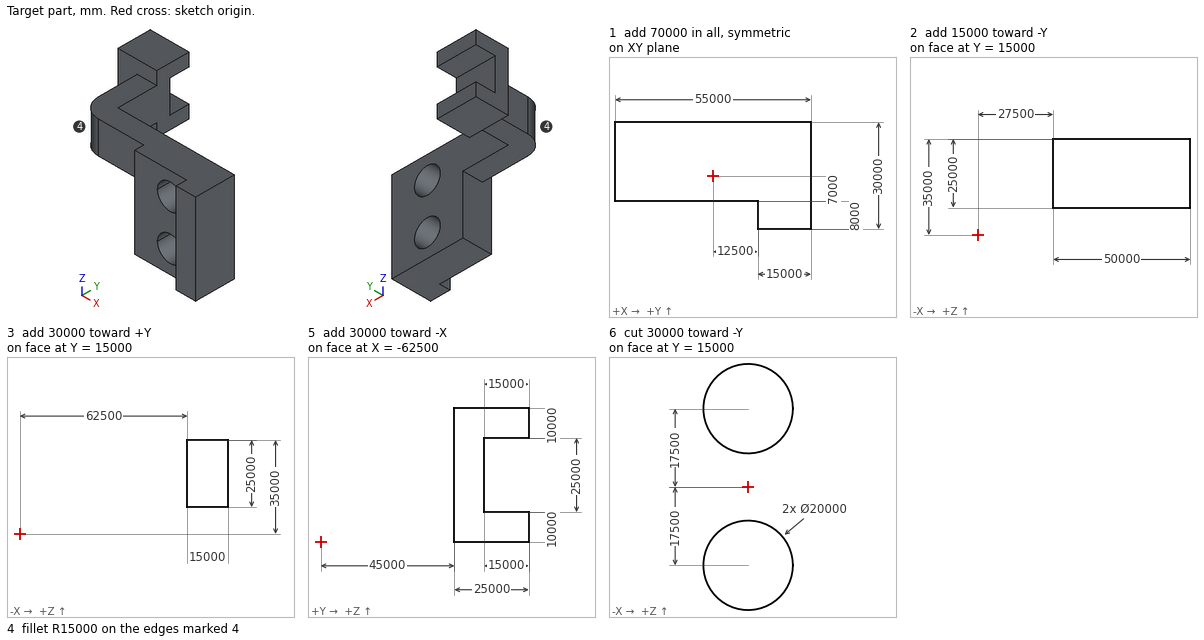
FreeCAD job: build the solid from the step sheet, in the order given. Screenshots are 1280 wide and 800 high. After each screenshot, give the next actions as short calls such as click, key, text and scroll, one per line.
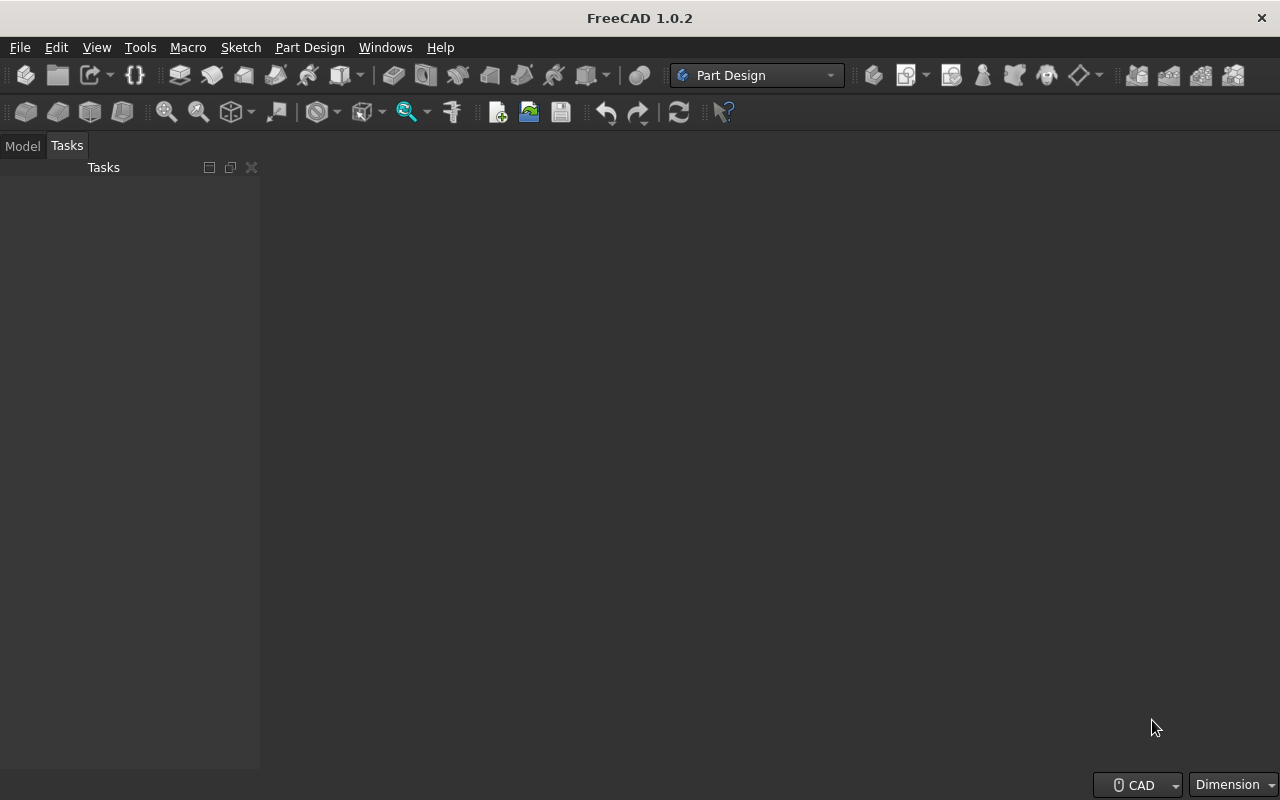
key(ctrl+n)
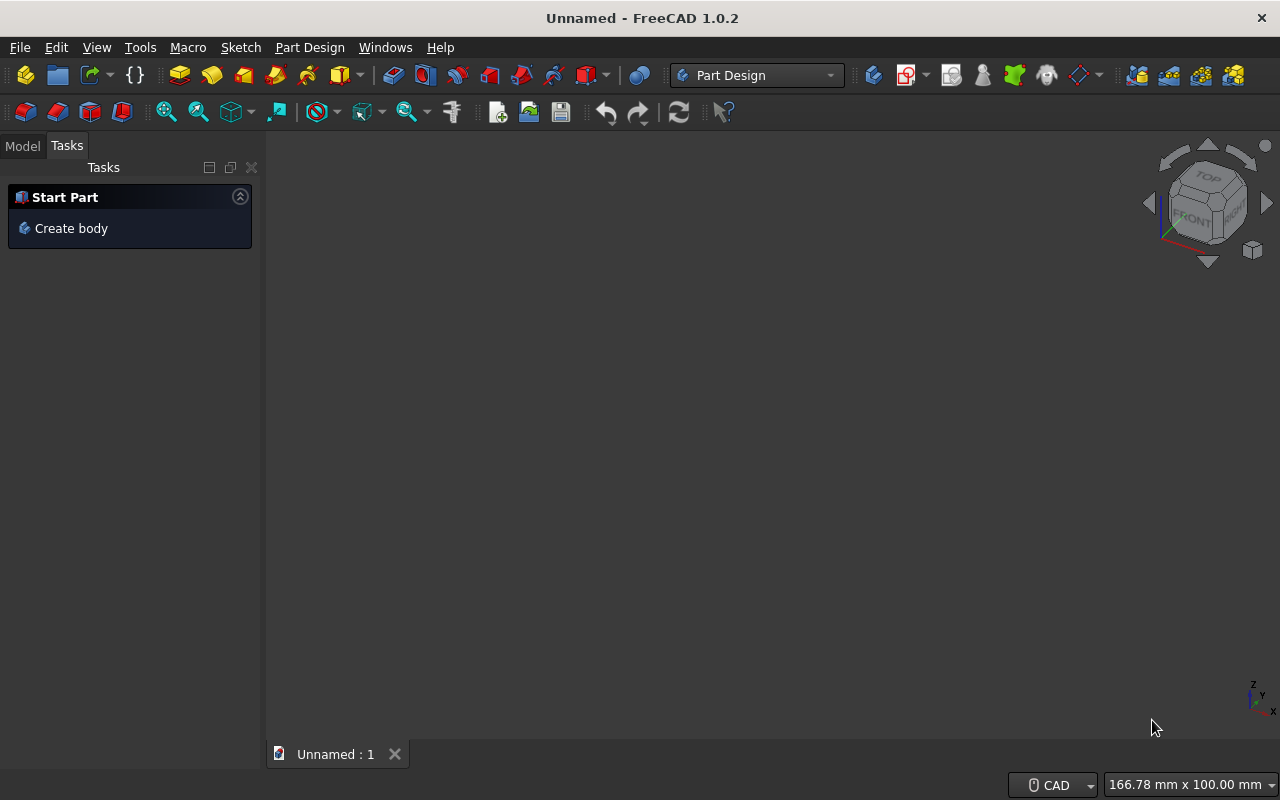
click(906, 76)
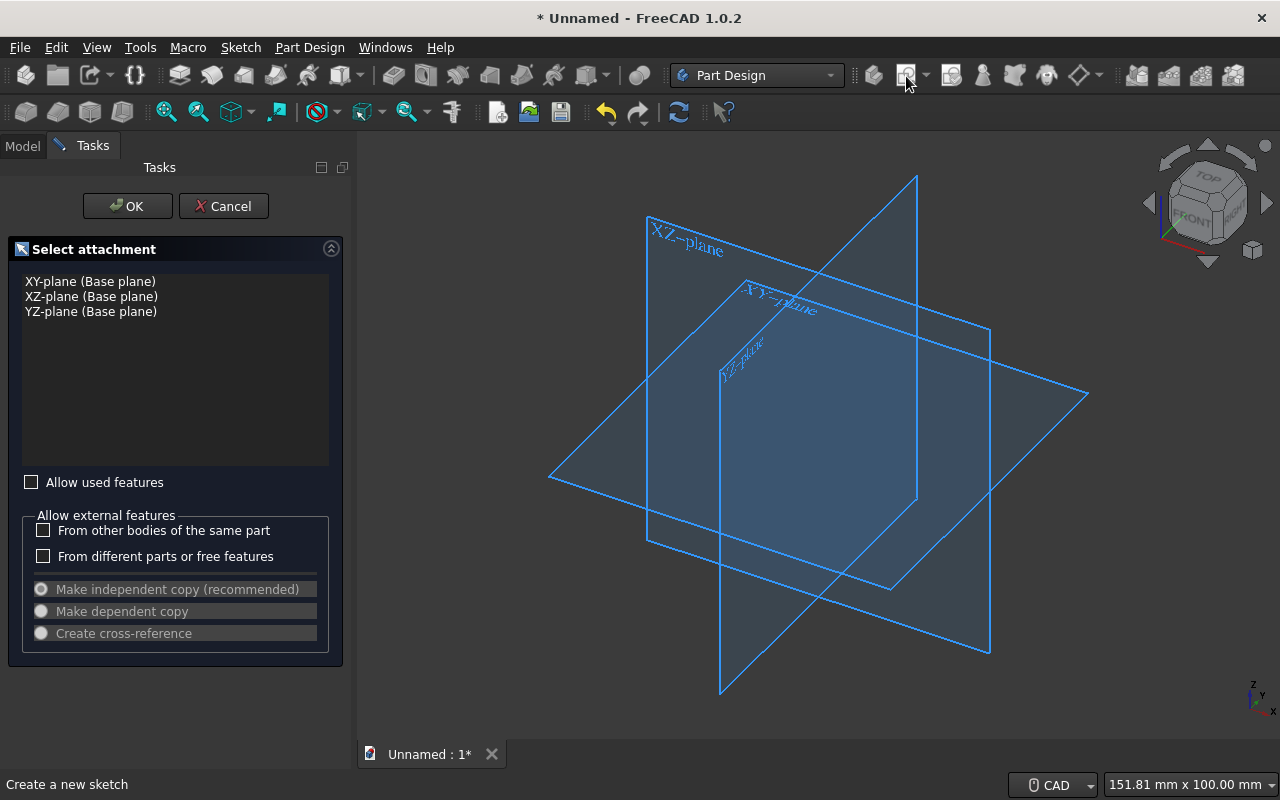
click(82, 282)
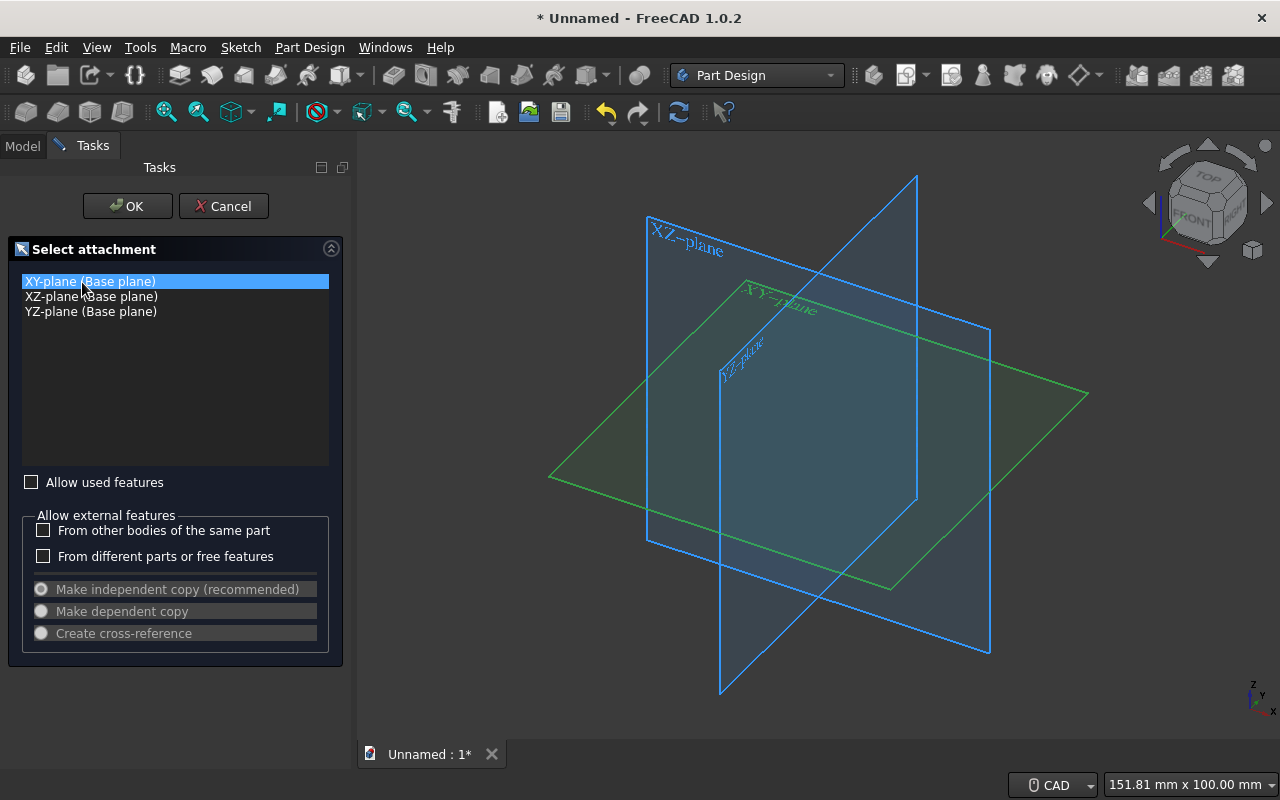
click(128, 206)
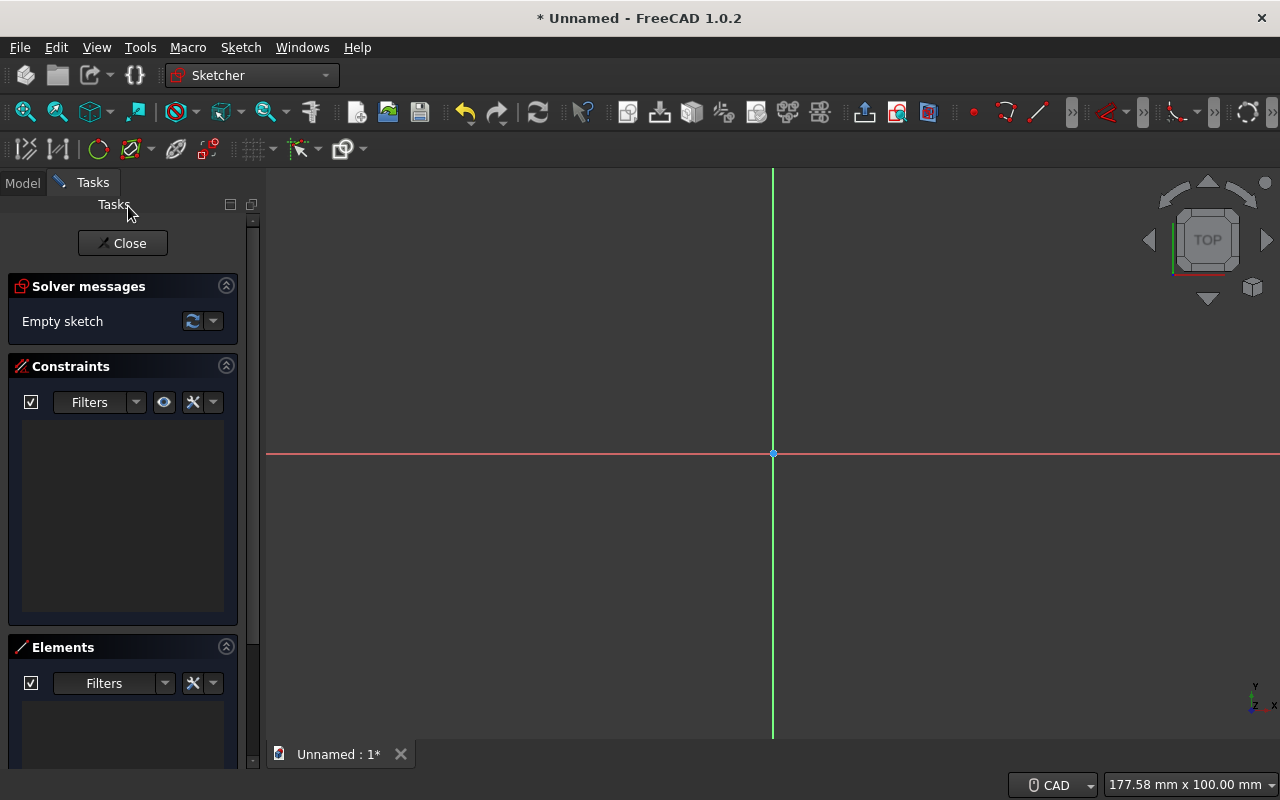
scroll(704, 454, down, 15)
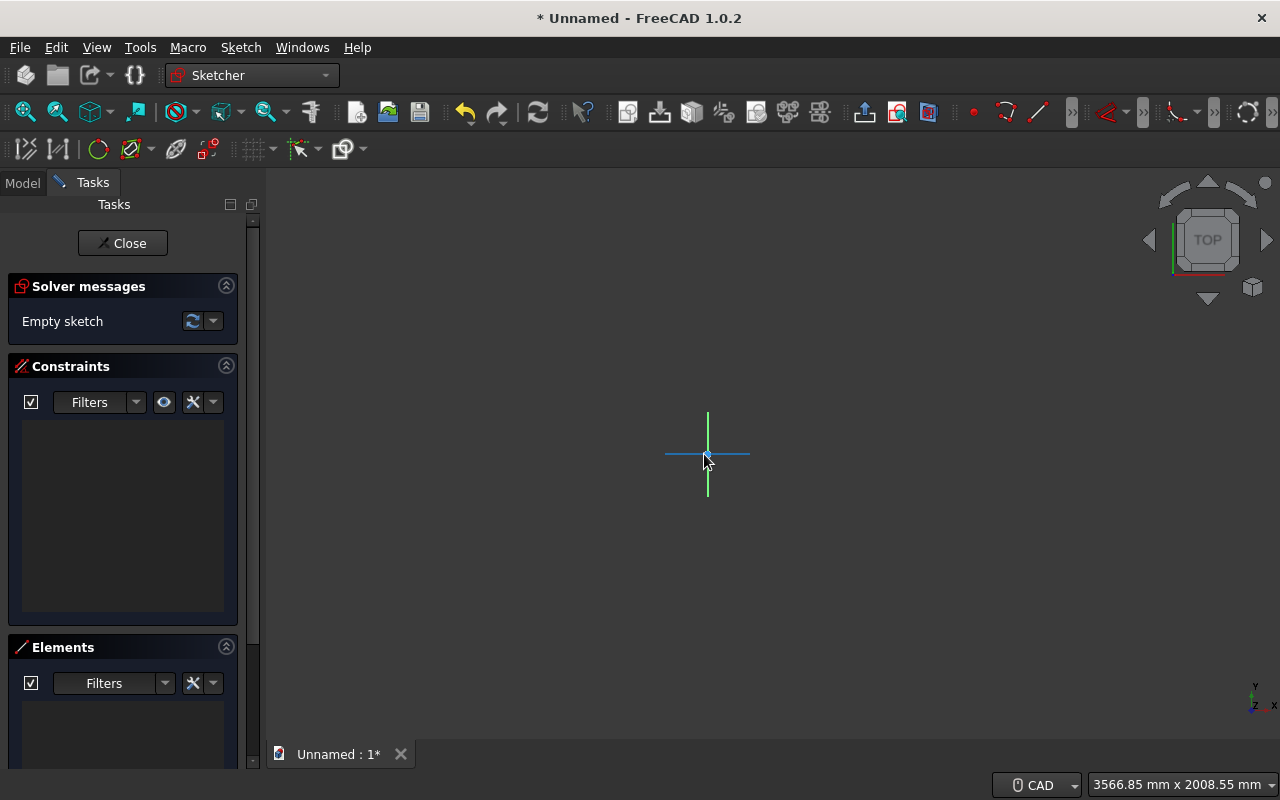
scroll(704, 453, down, 16)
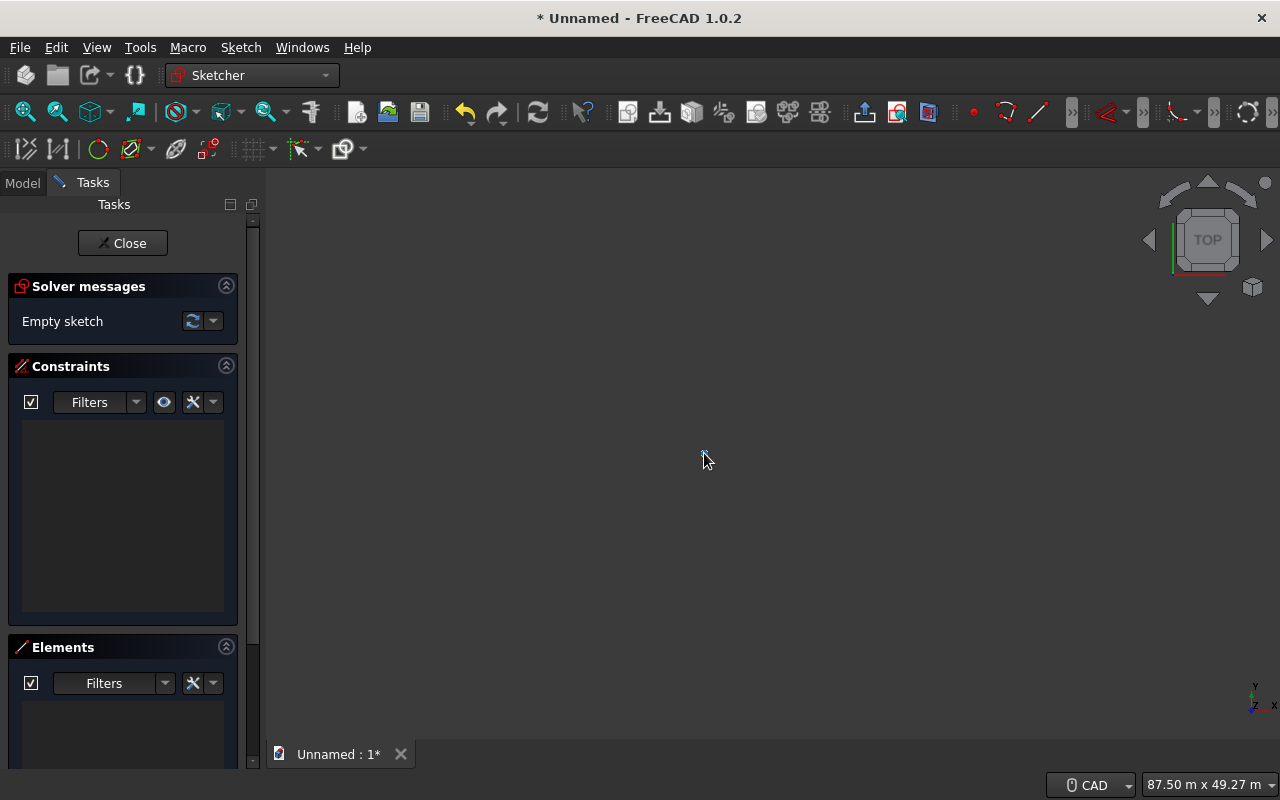
click(1006, 112)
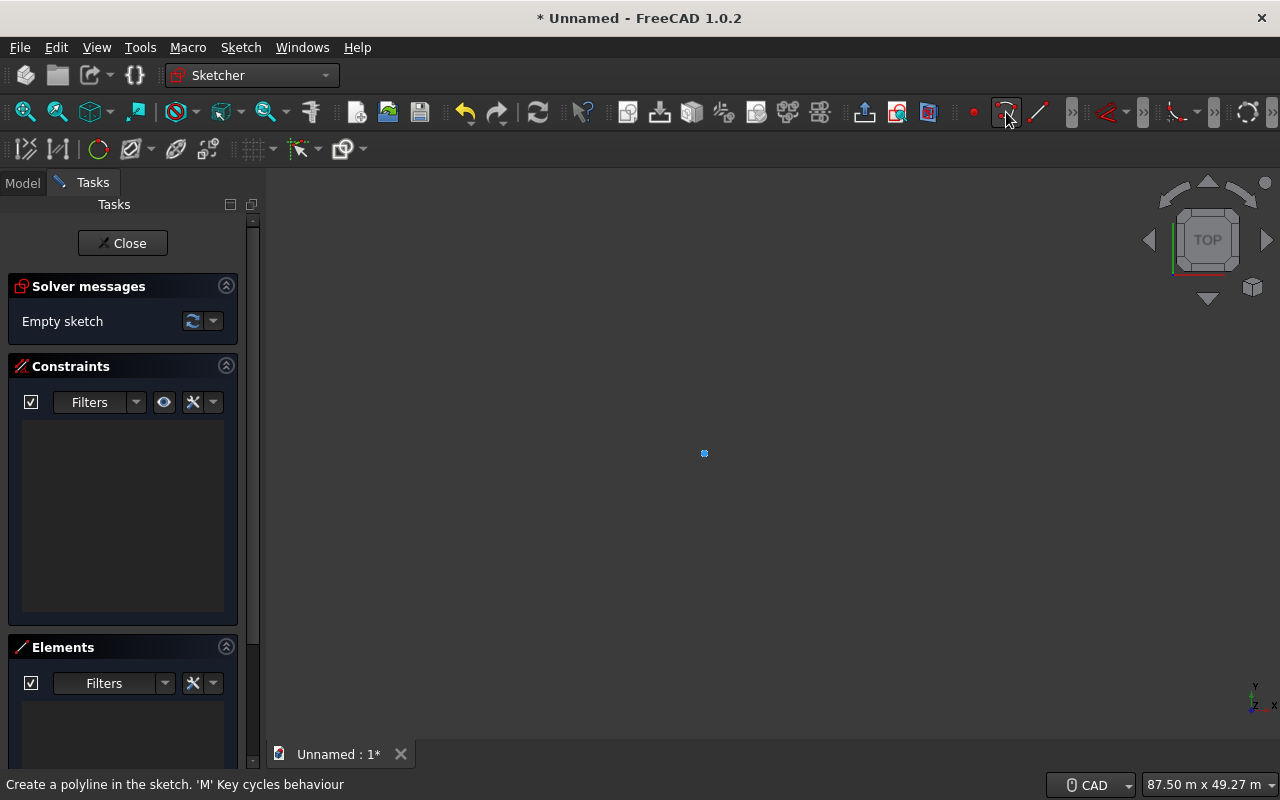
click(849, 535)
click(849, 627)
click(1023, 627)
click(1023, 280)
click(386, 280)
click(386, 535)
click(849, 536)
key(Escape)
key(Escape)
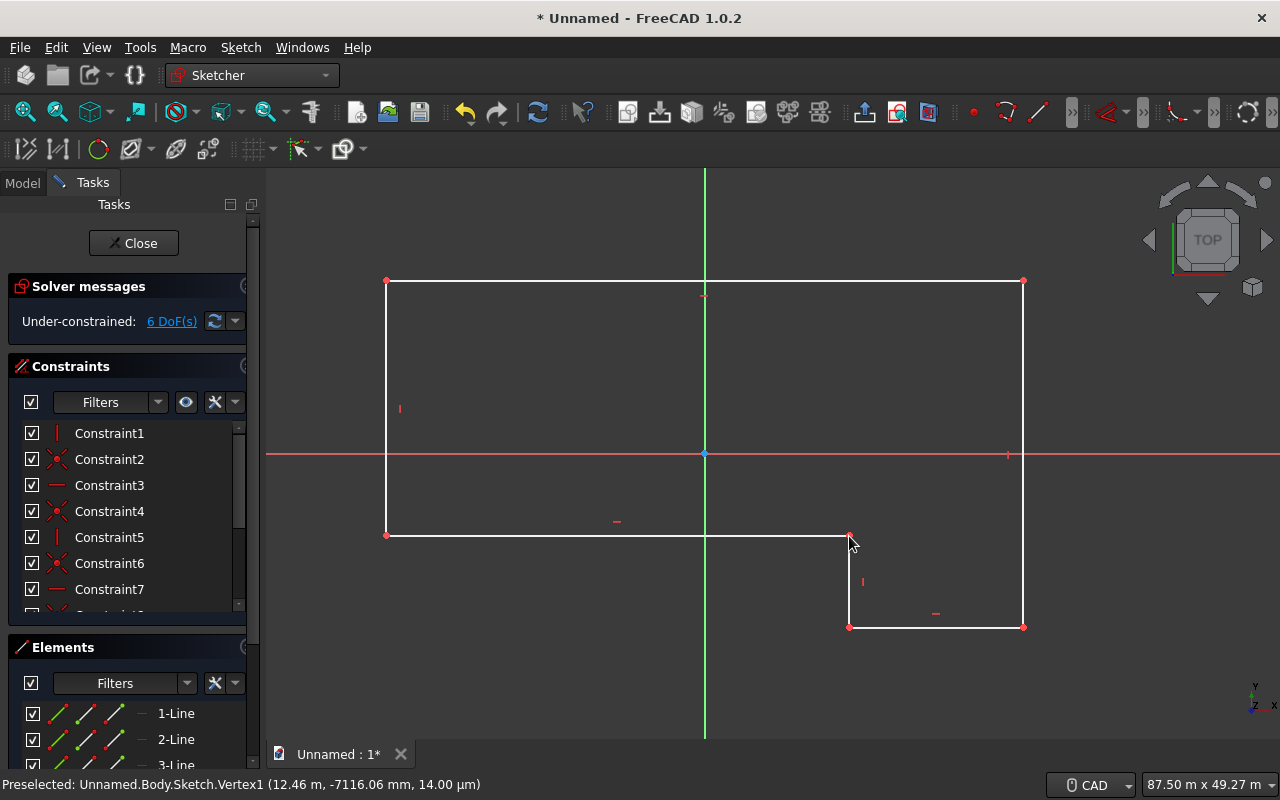
key(d)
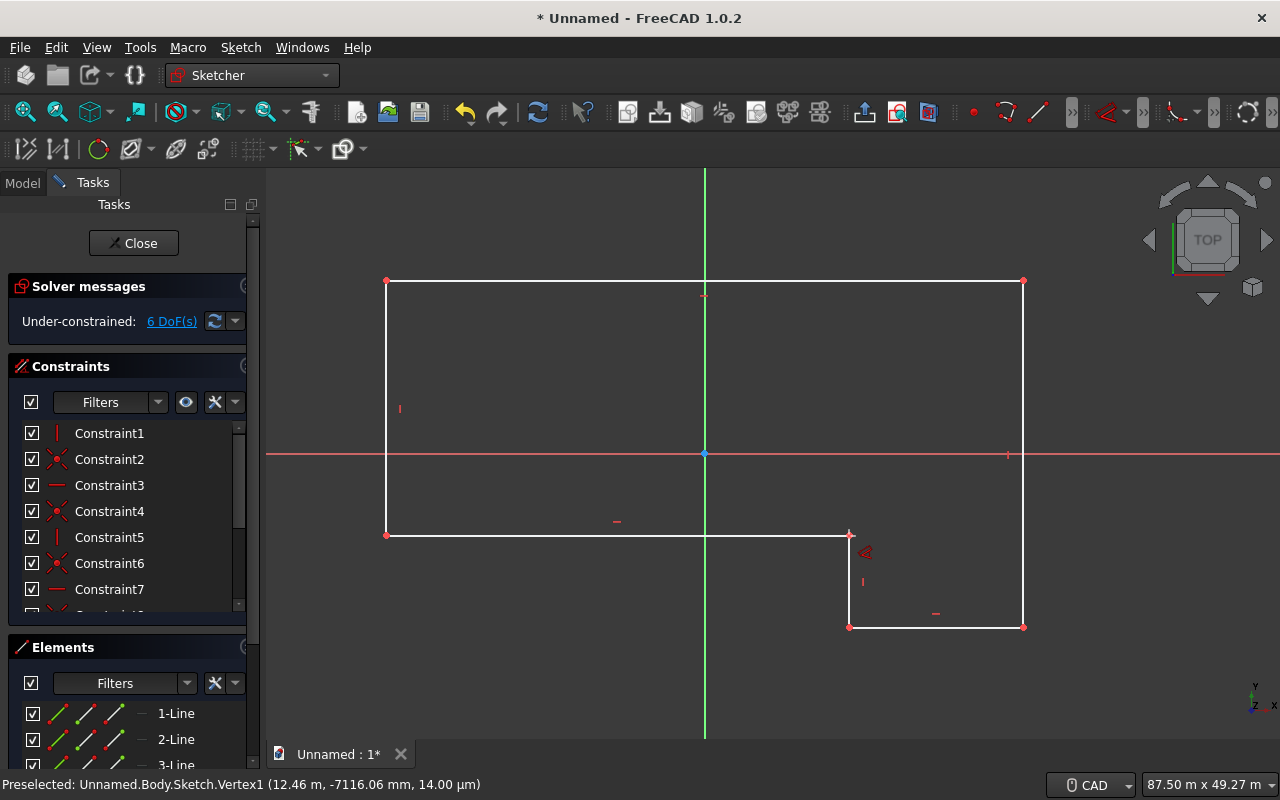
click(849, 564)
click(883, 582)